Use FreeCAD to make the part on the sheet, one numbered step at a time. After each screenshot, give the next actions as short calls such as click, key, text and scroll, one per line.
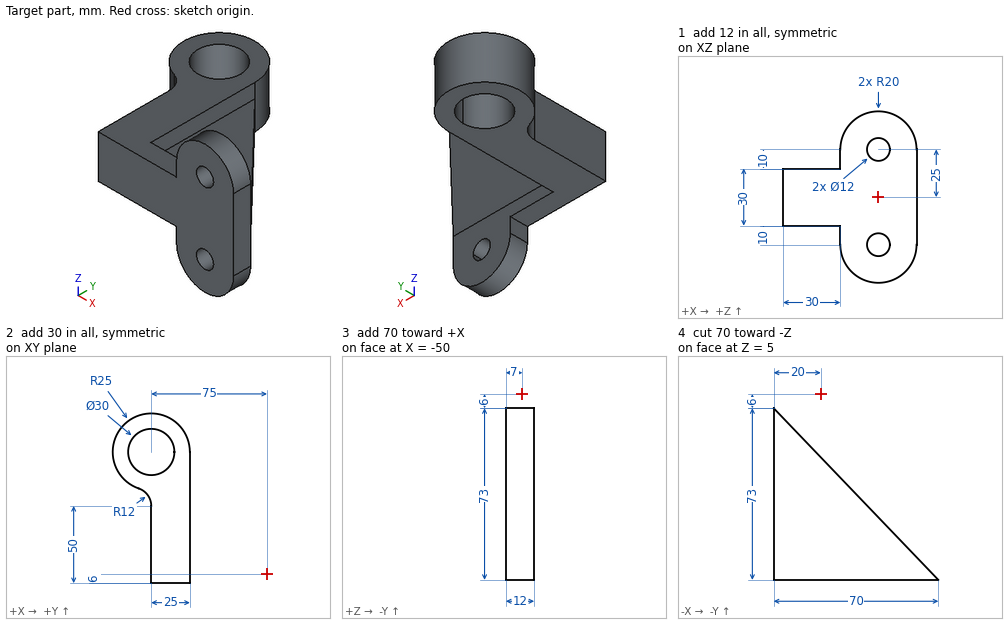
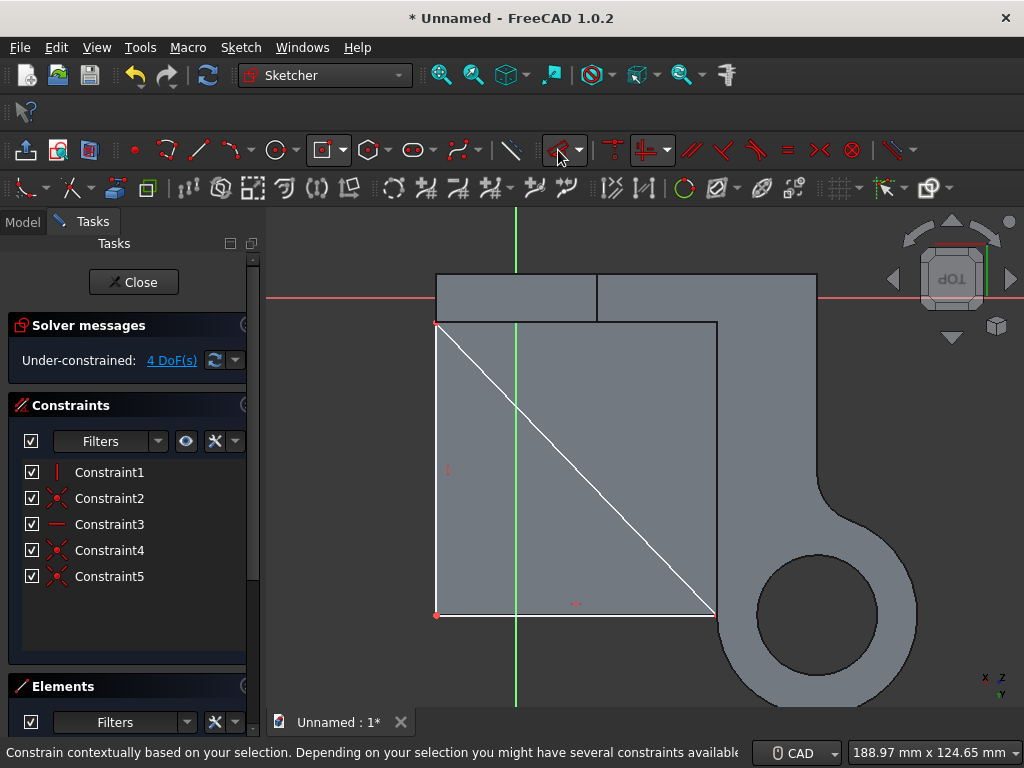
click(436, 411)
click(402, 470)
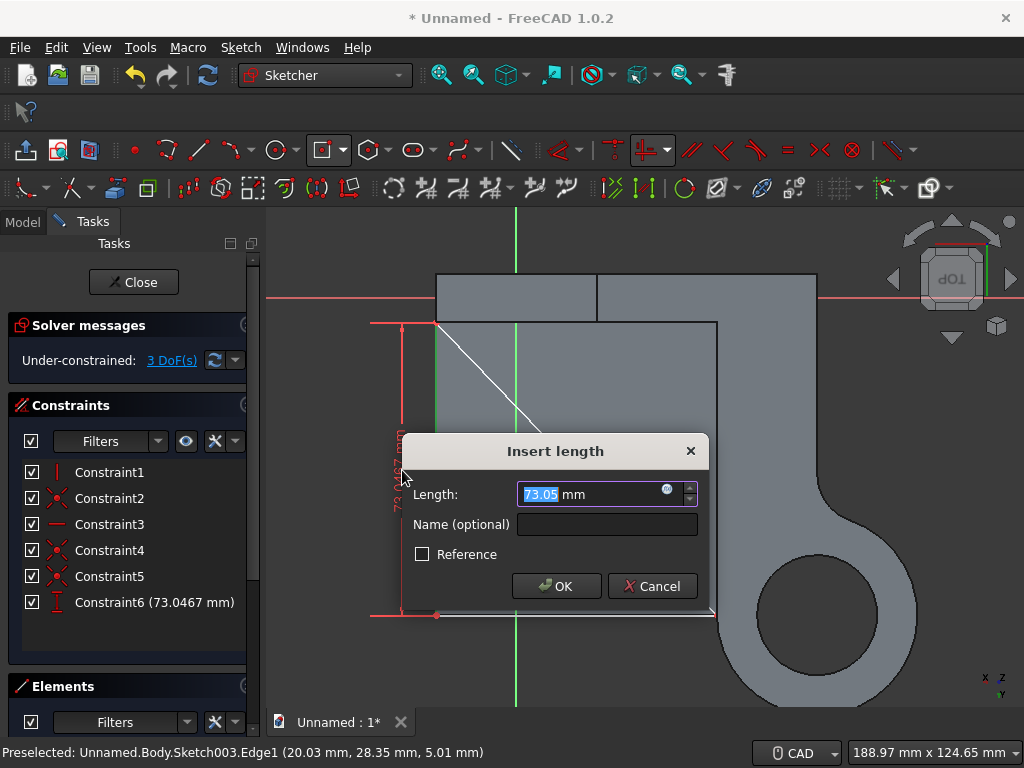
text(73)
key(Return)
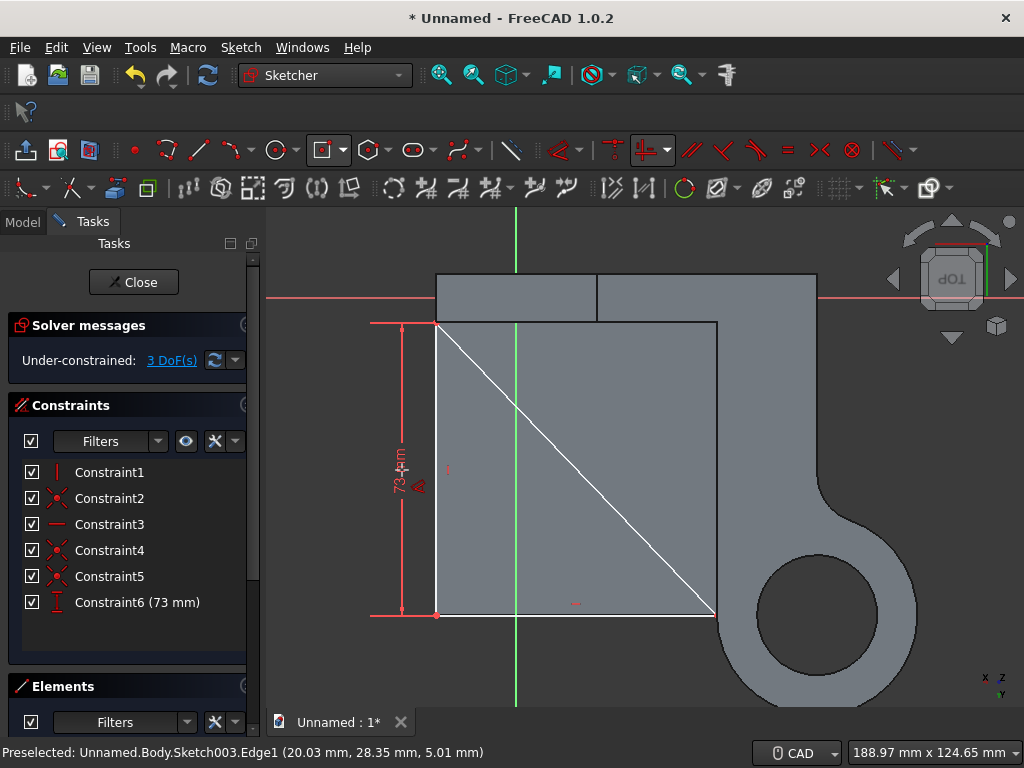
click(520, 616)
click(576, 650)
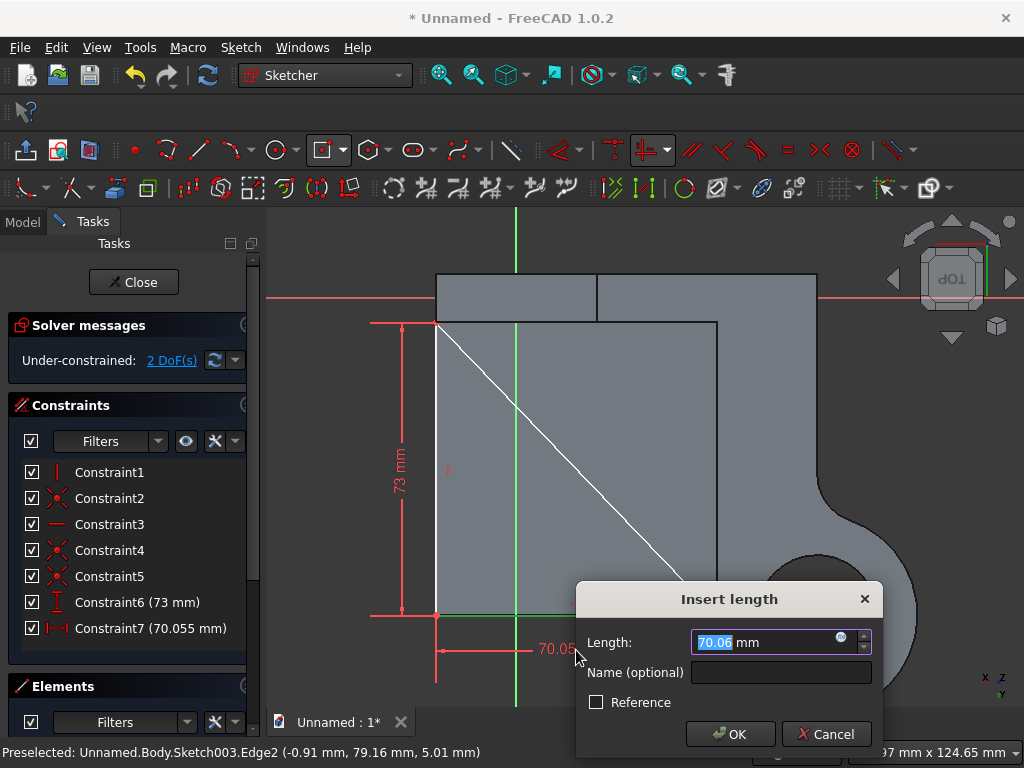
text(70)
key(Return)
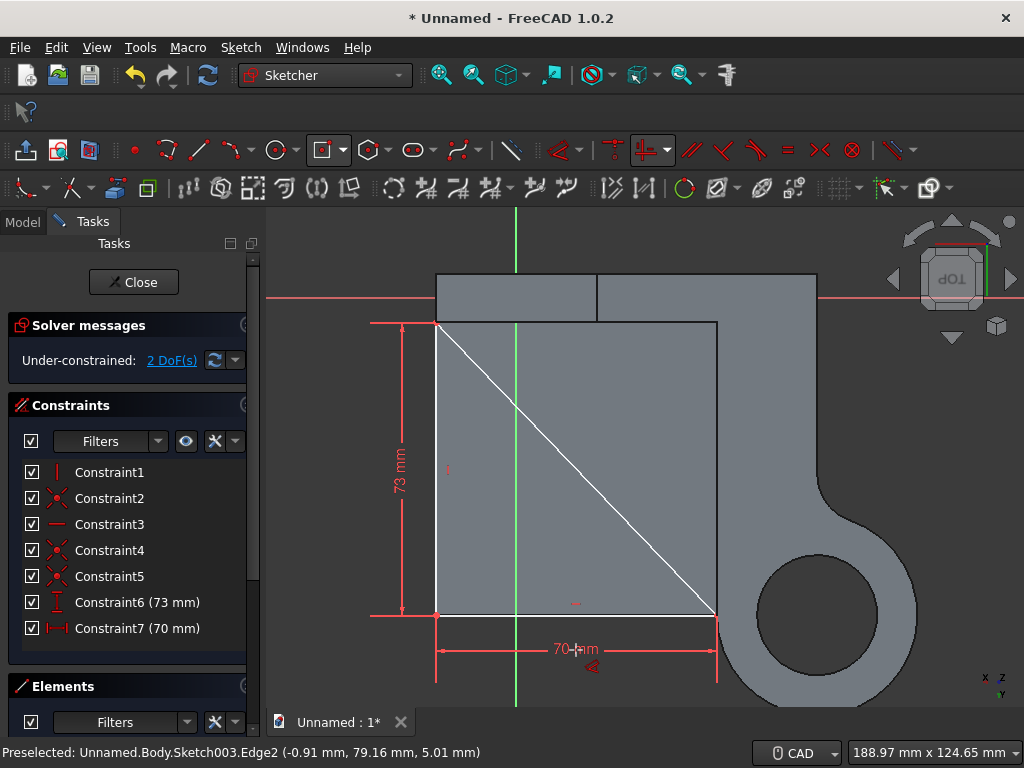
scroll(436, 323, up, 3)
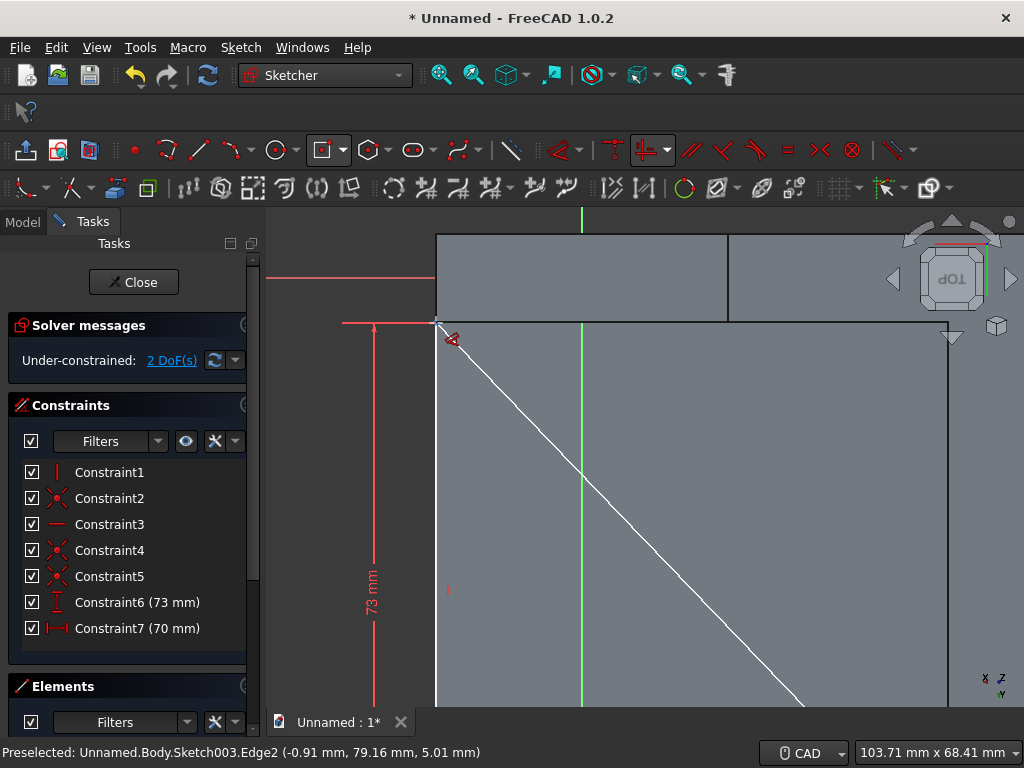
click(436, 323)
click(402, 300)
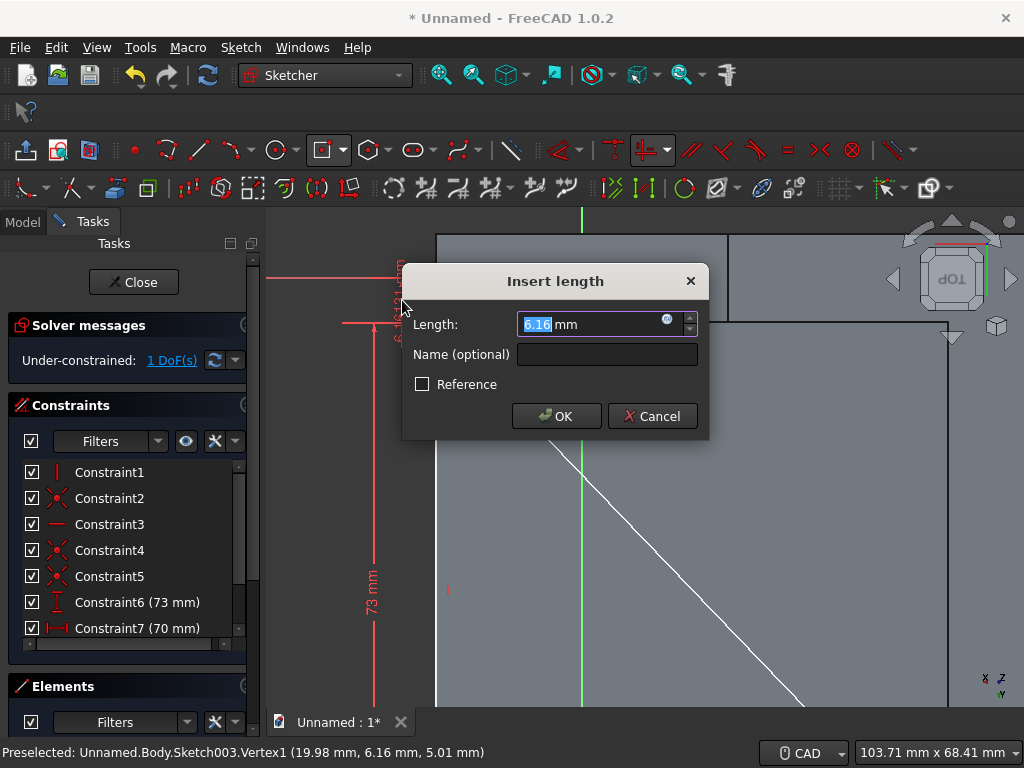
text(6)
key(Return)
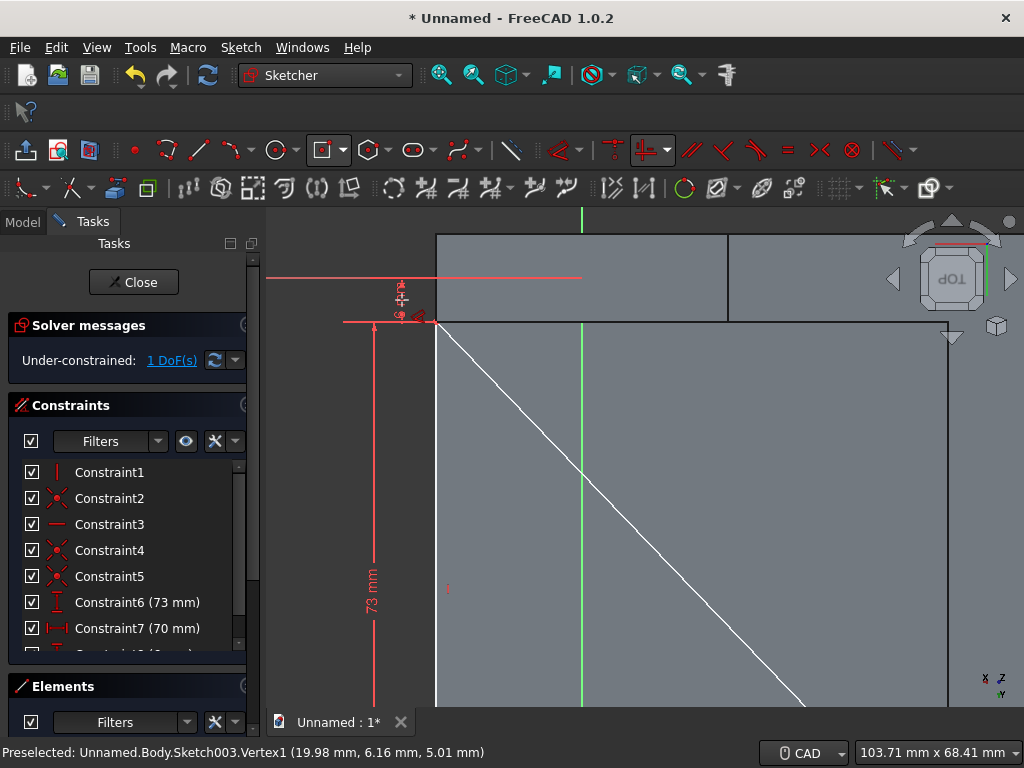
click(436, 322)
click(509, 244)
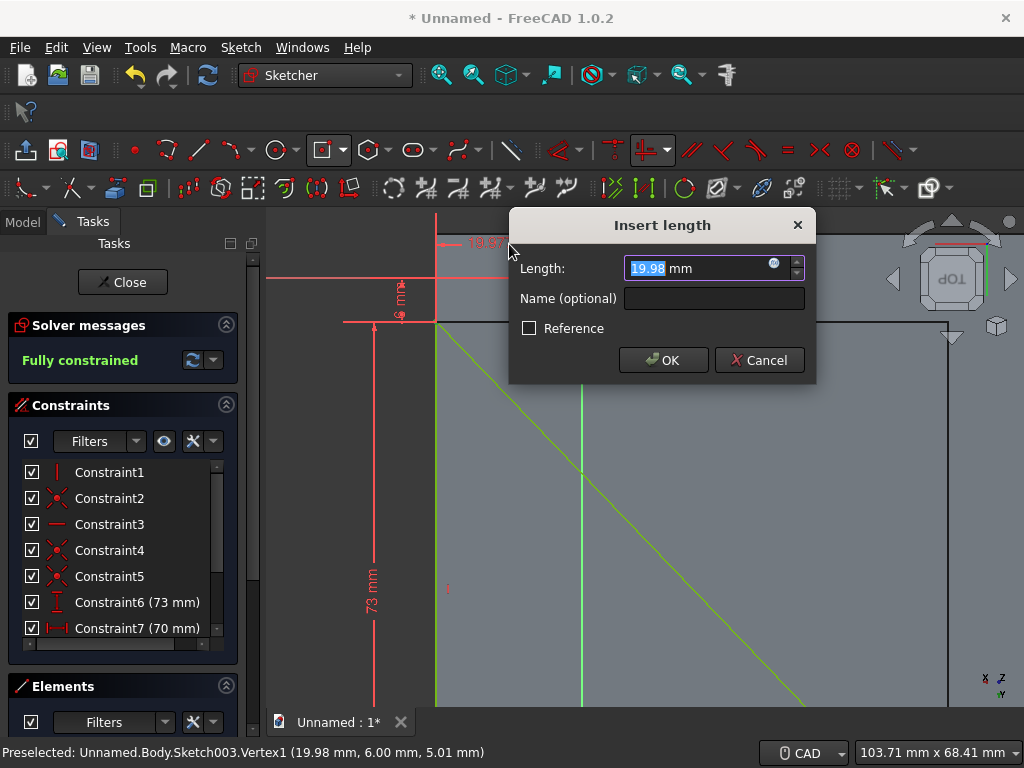
text(20)
key(Return)
key(Escape)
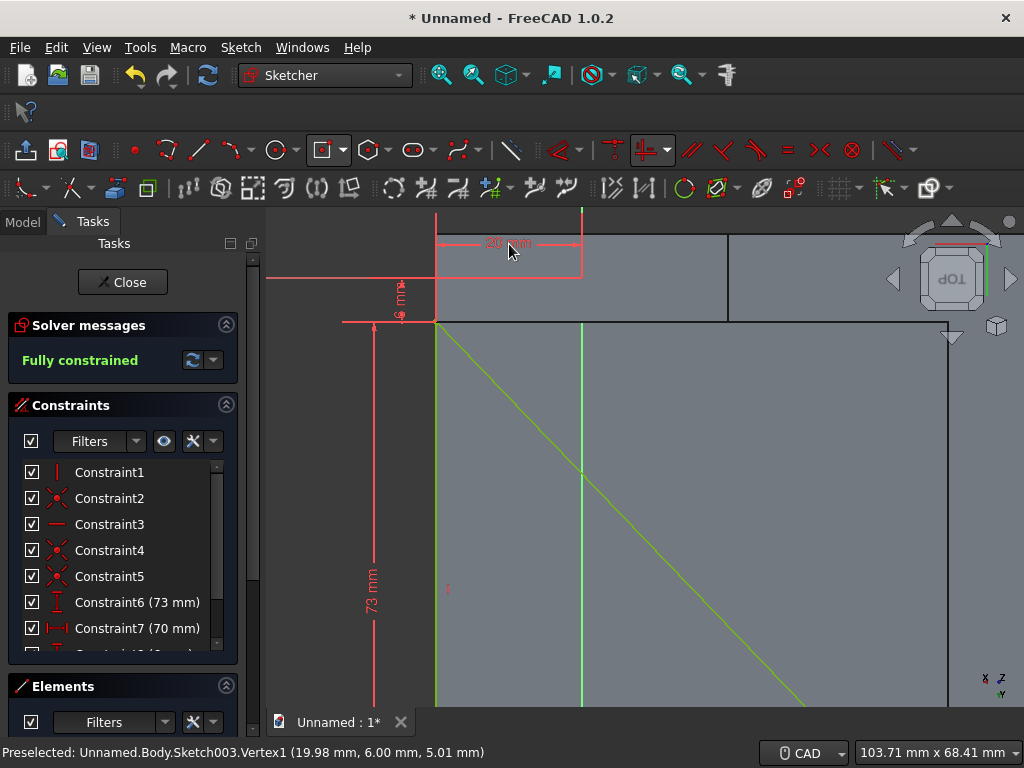
click(123, 282)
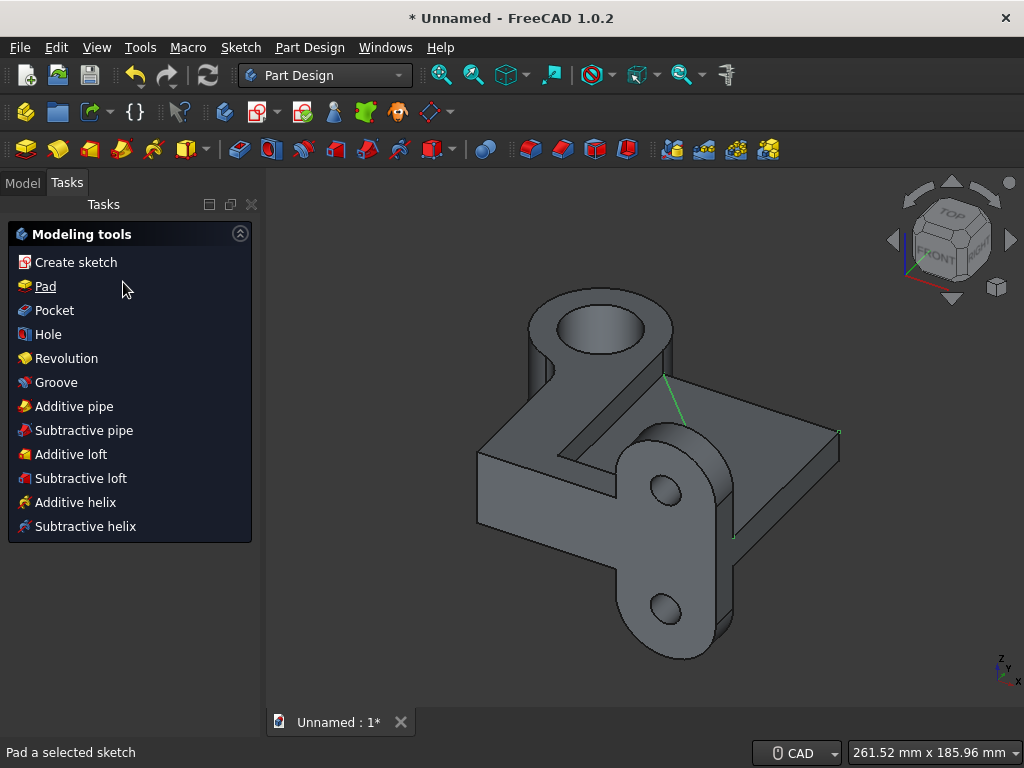
click(240, 150)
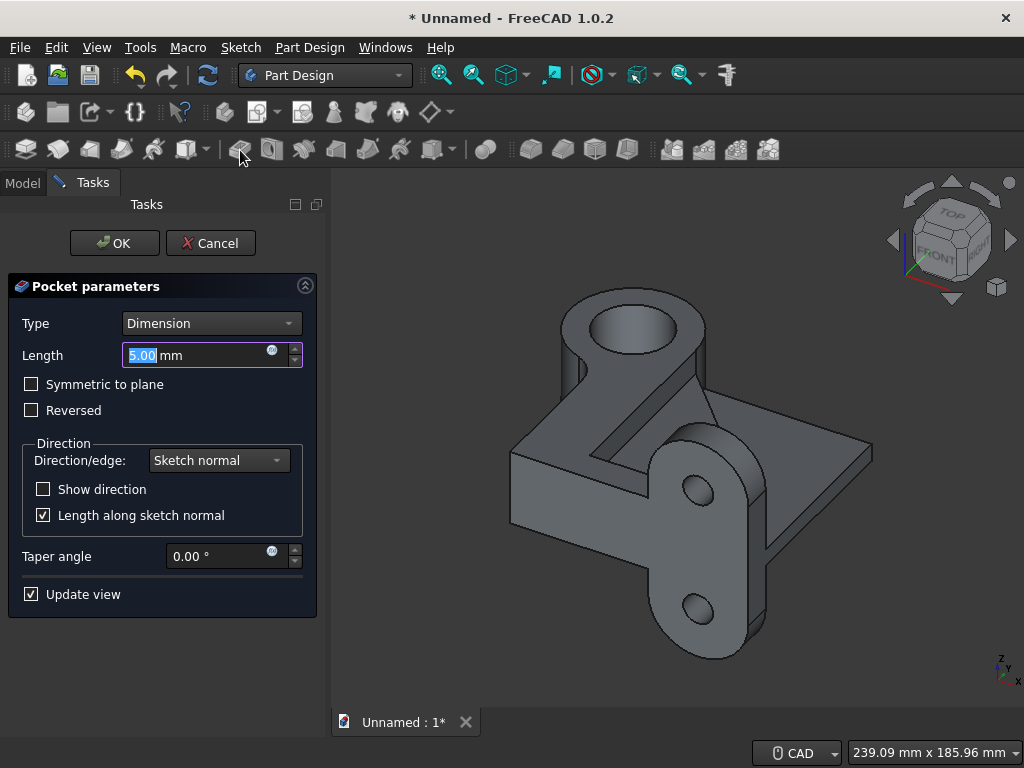
text(70)
key(Tab)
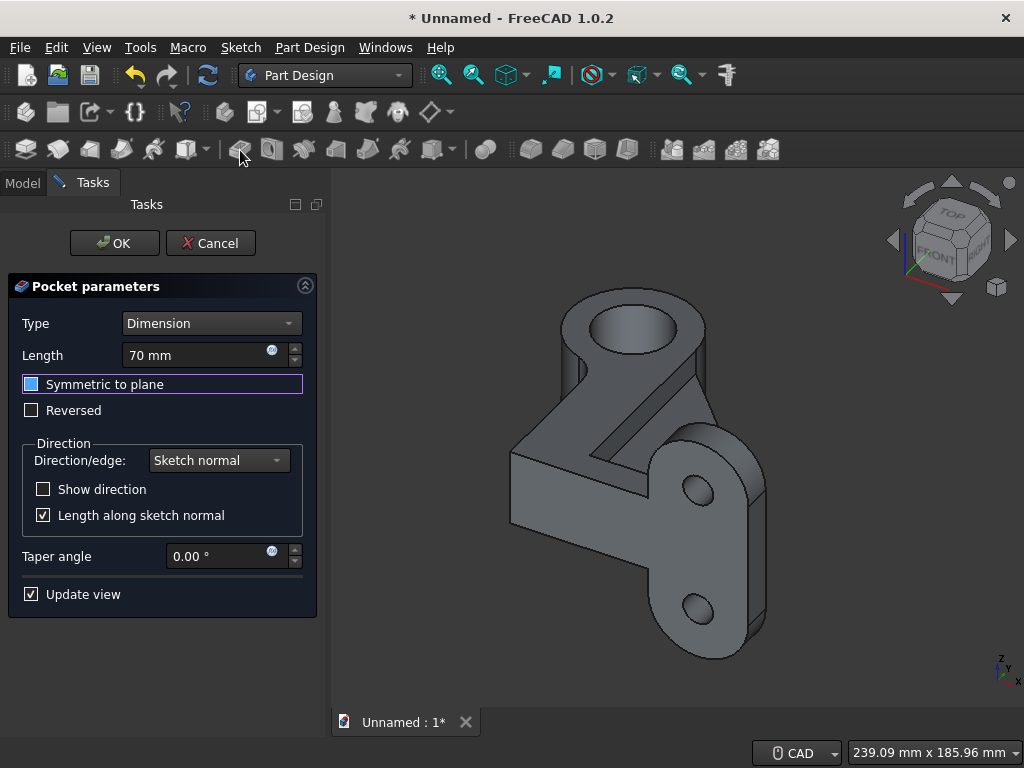
click(115, 243)